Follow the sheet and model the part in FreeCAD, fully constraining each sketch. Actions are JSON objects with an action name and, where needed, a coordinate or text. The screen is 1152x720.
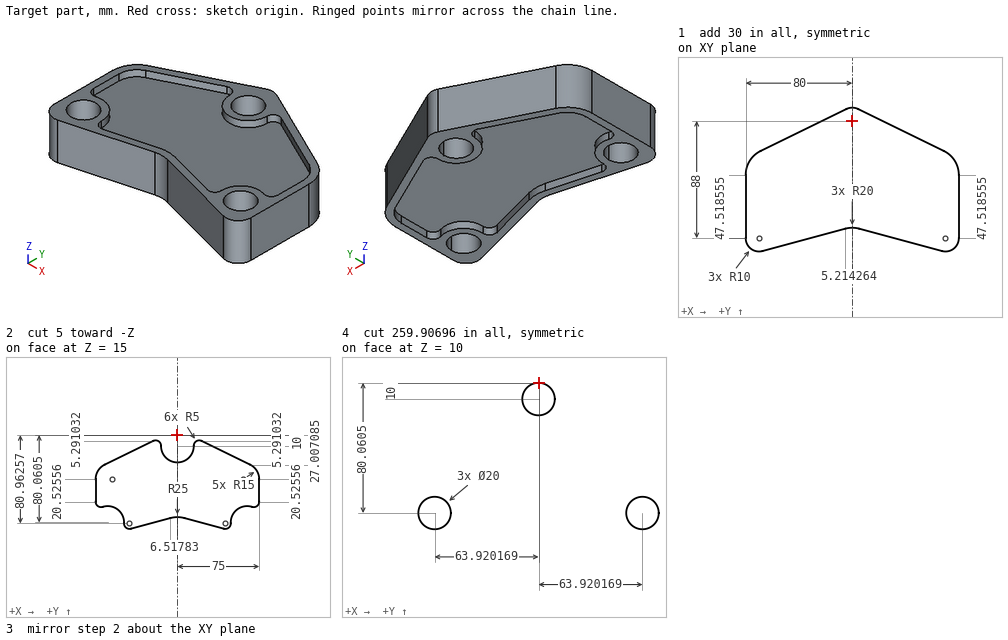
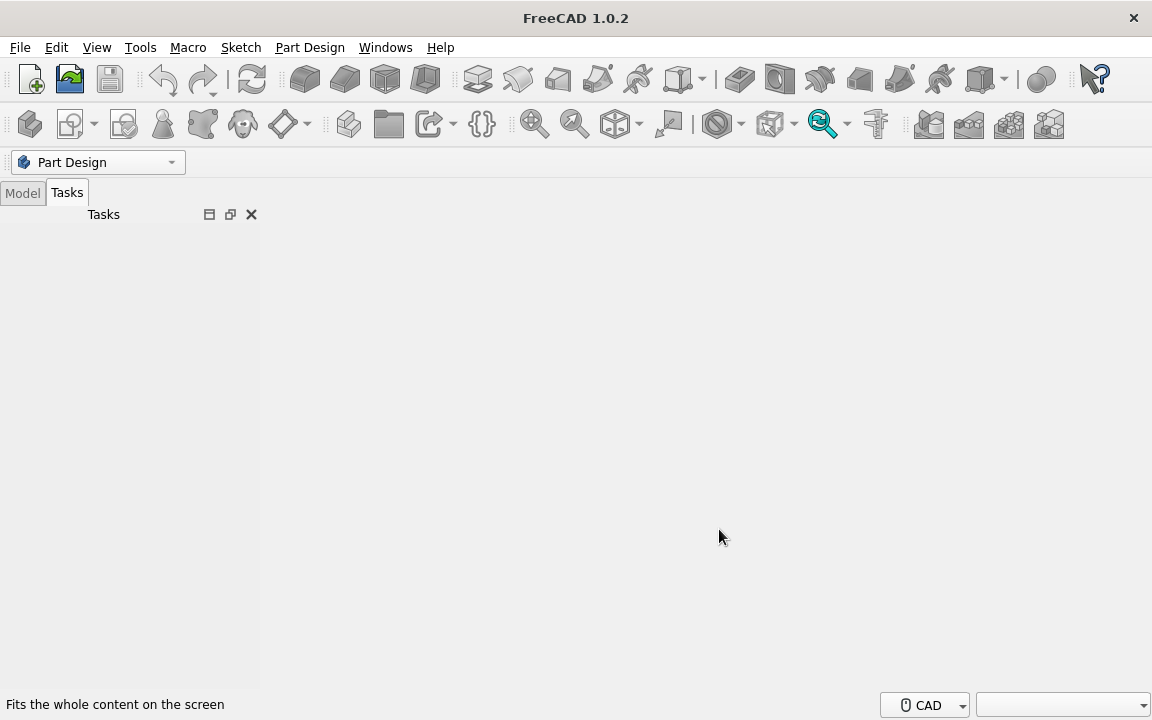
{"action": "left_click", "coordinate": [30, 80]}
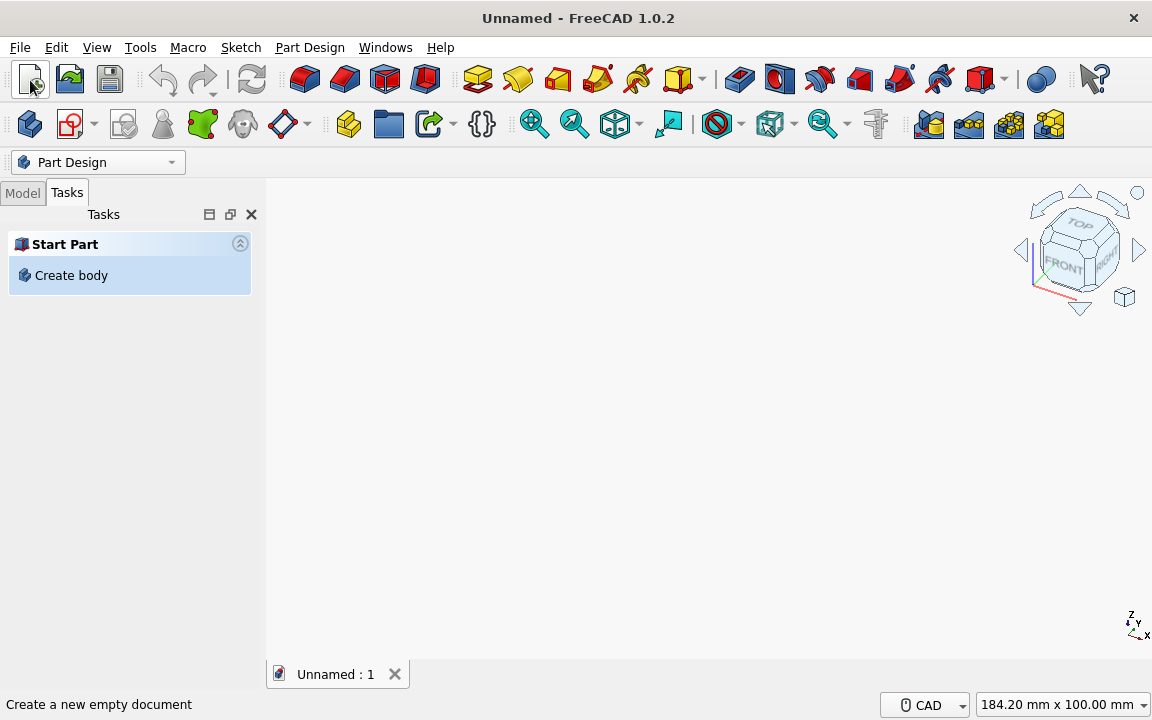
{"action": "left_click", "coordinate": [70, 124]}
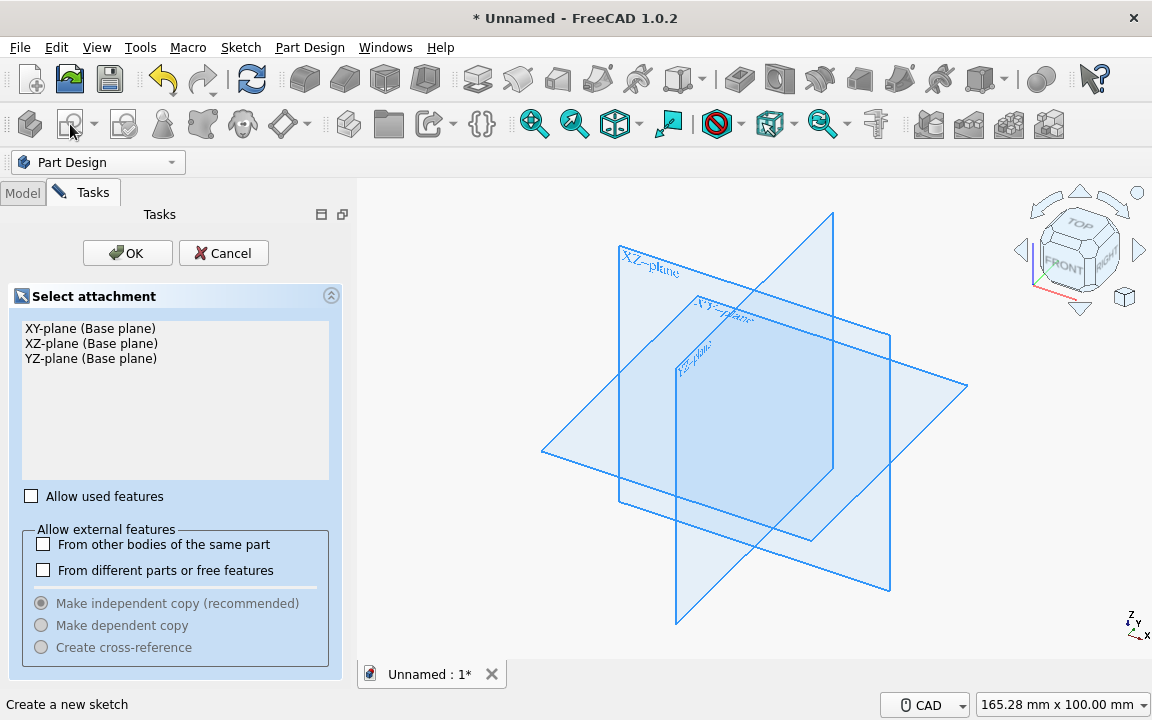
{"action": "left_click", "coordinate": [82, 328]}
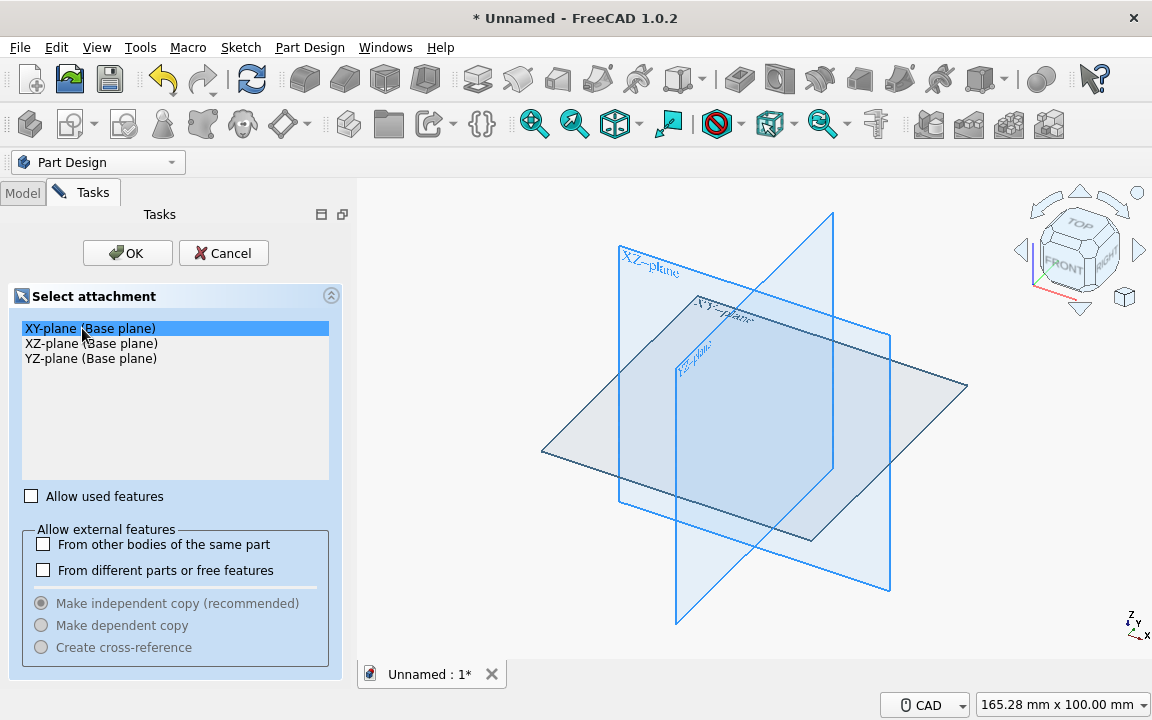
{"action": "left_click", "coordinate": [128, 253]}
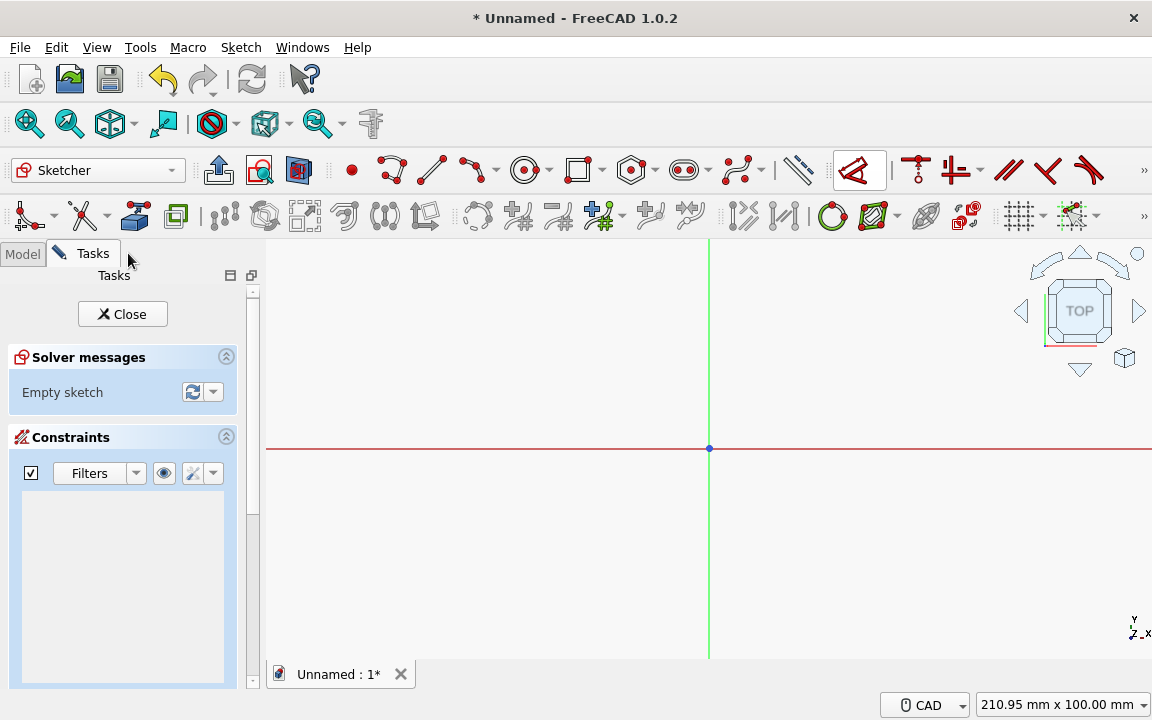
{"action": "scroll", "coordinate": [557, 267], "scroll_direction": "down", "scroll_amount": 3}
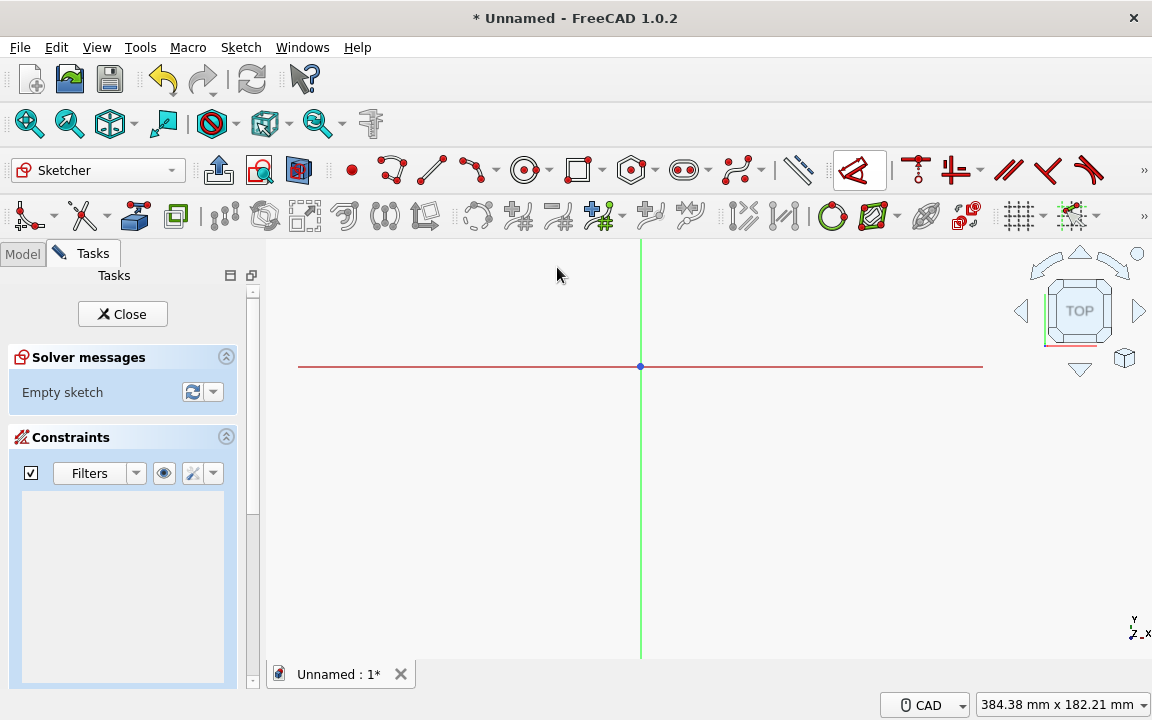
{"action": "left_click", "coordinate": [432, 170]}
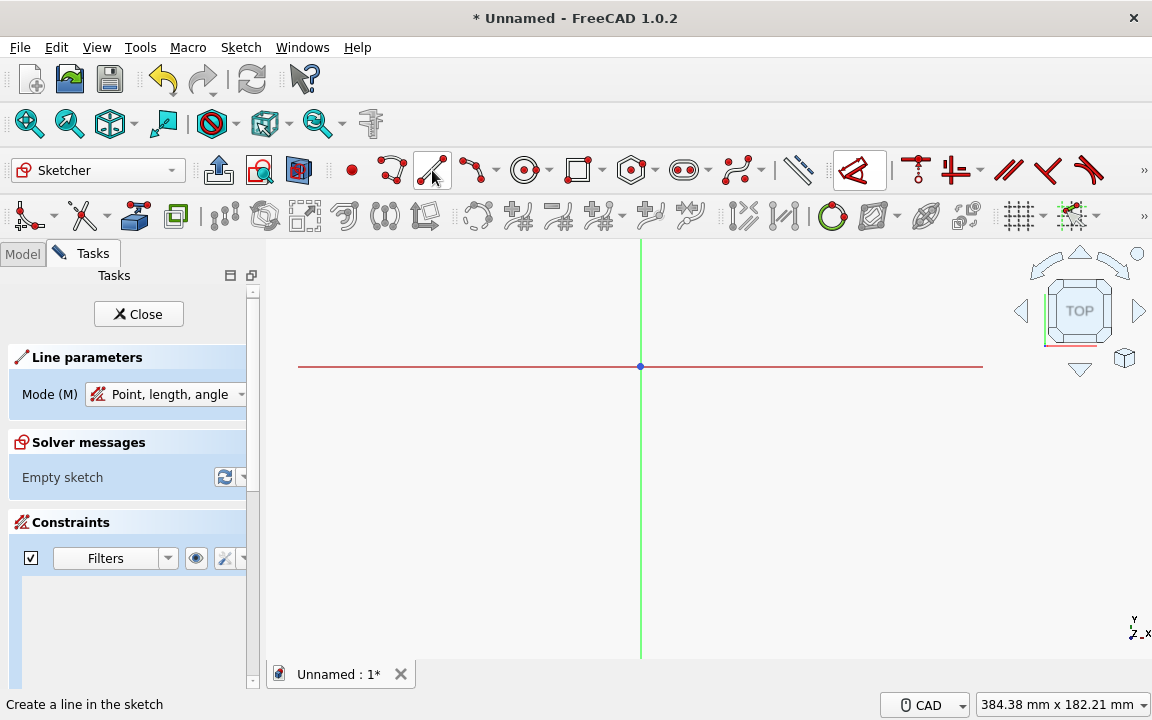
{"action": "left_click", "coordinate": [456, 460]}
{"action": "left_click", "coordinate": [456, 570]}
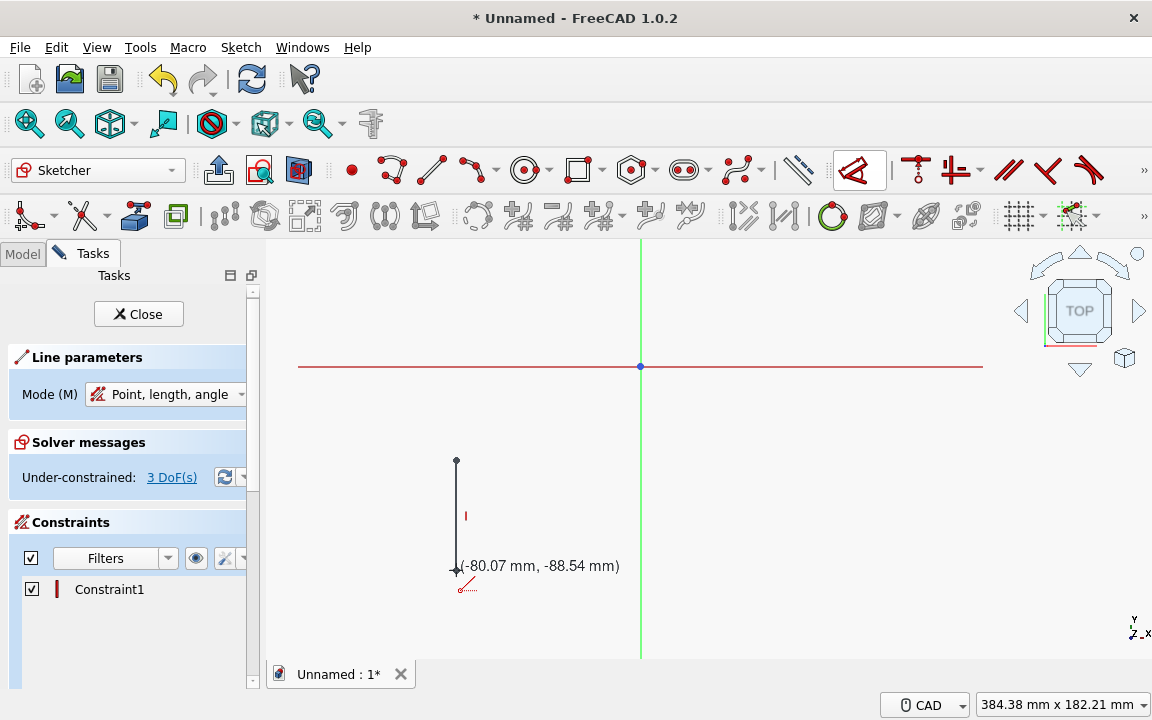
{"action": "left_click", "coordinate": [485, 592]}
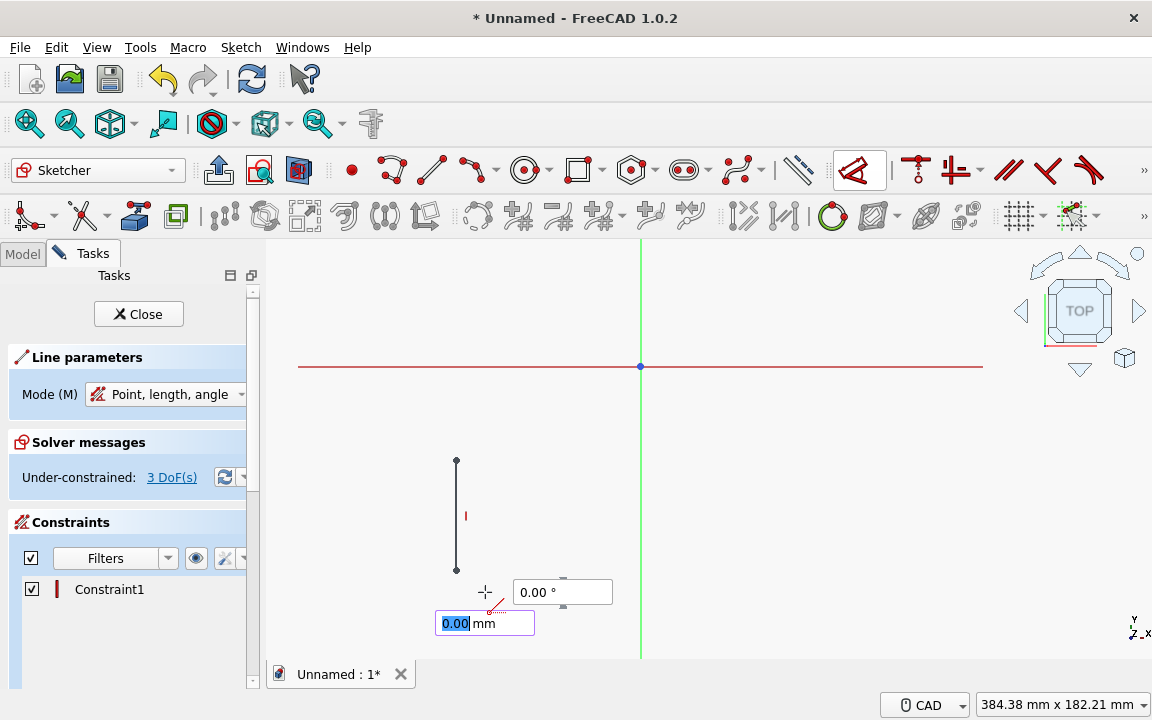
{"action": "scroll", "coordinate": [629, 553], "scroll_direction": "up", "scroll_amount": 2}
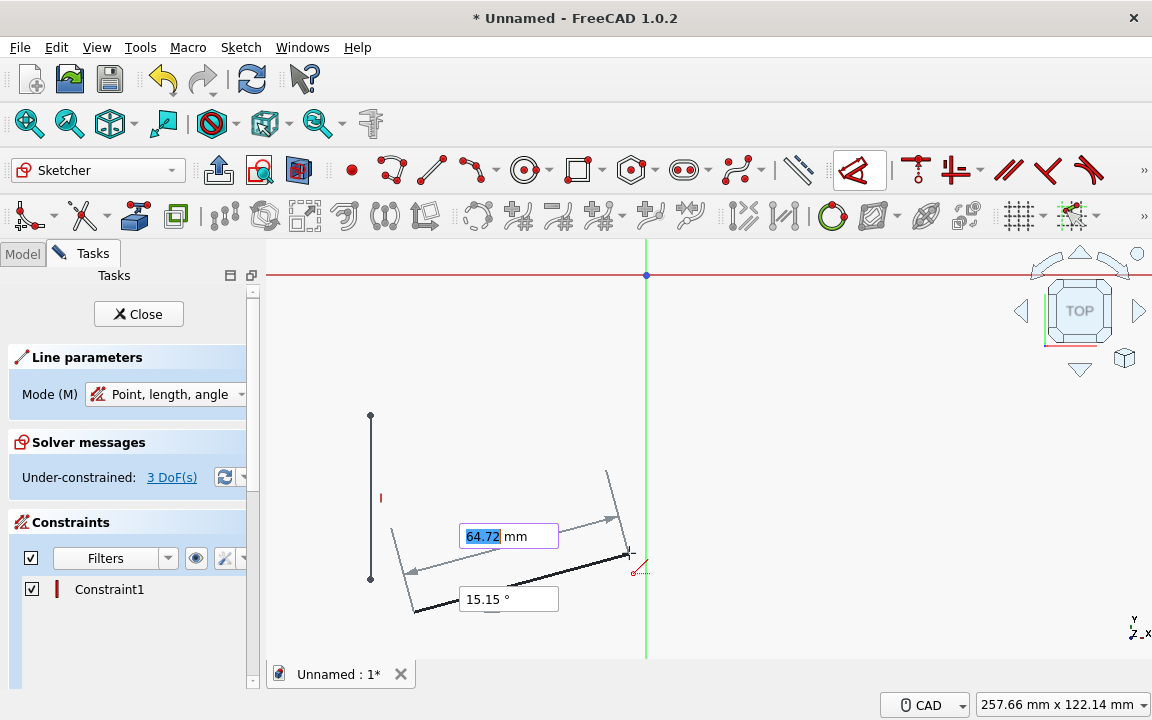
{"action": "left_click", "coordinate": [628, 553]}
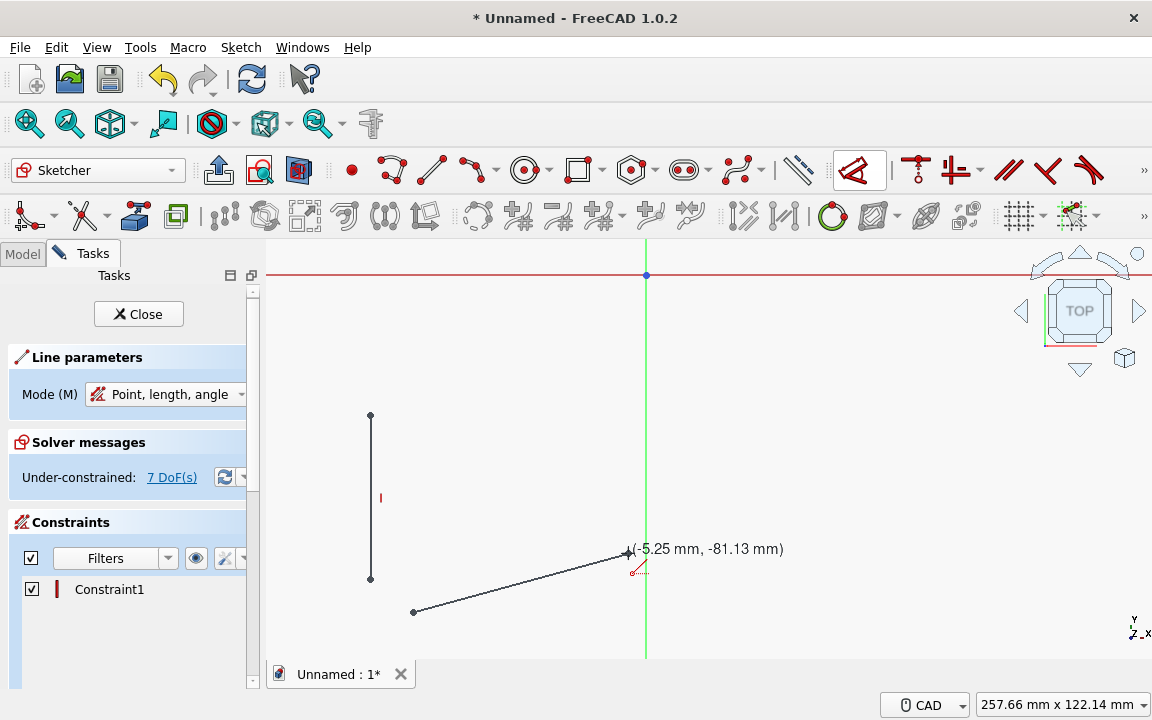
{"action": "left_click", "coordinate": [664, 553]}
{"action": "left_click", "coordinate": [878, 611]}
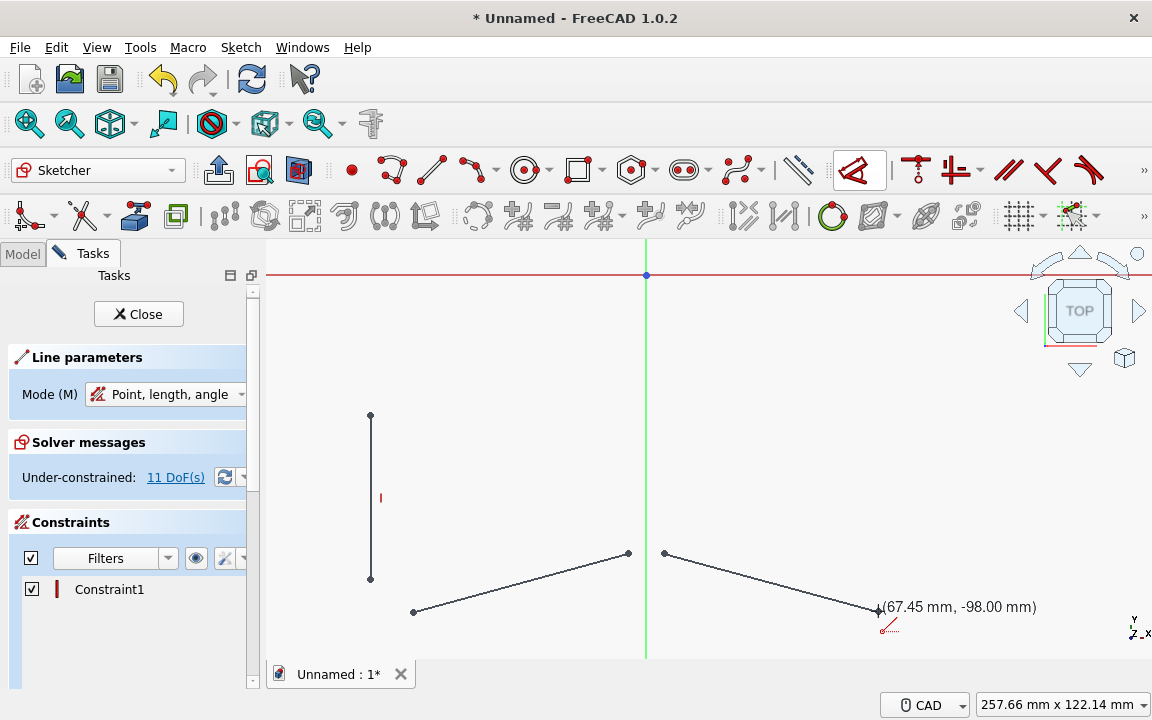
{"action": "left_click", "coordinate": [921, 578]}
{"action": "left_click", "coordinate": [921, 414]}